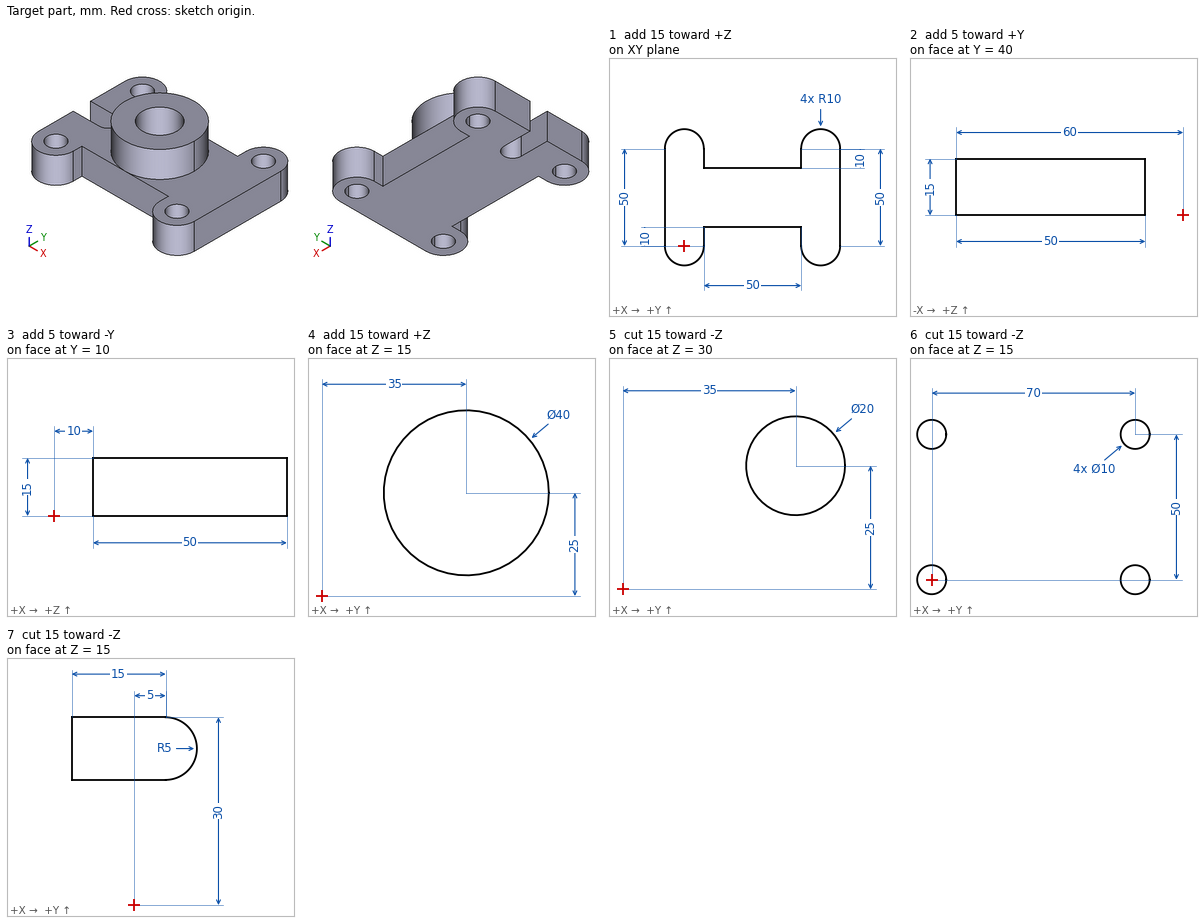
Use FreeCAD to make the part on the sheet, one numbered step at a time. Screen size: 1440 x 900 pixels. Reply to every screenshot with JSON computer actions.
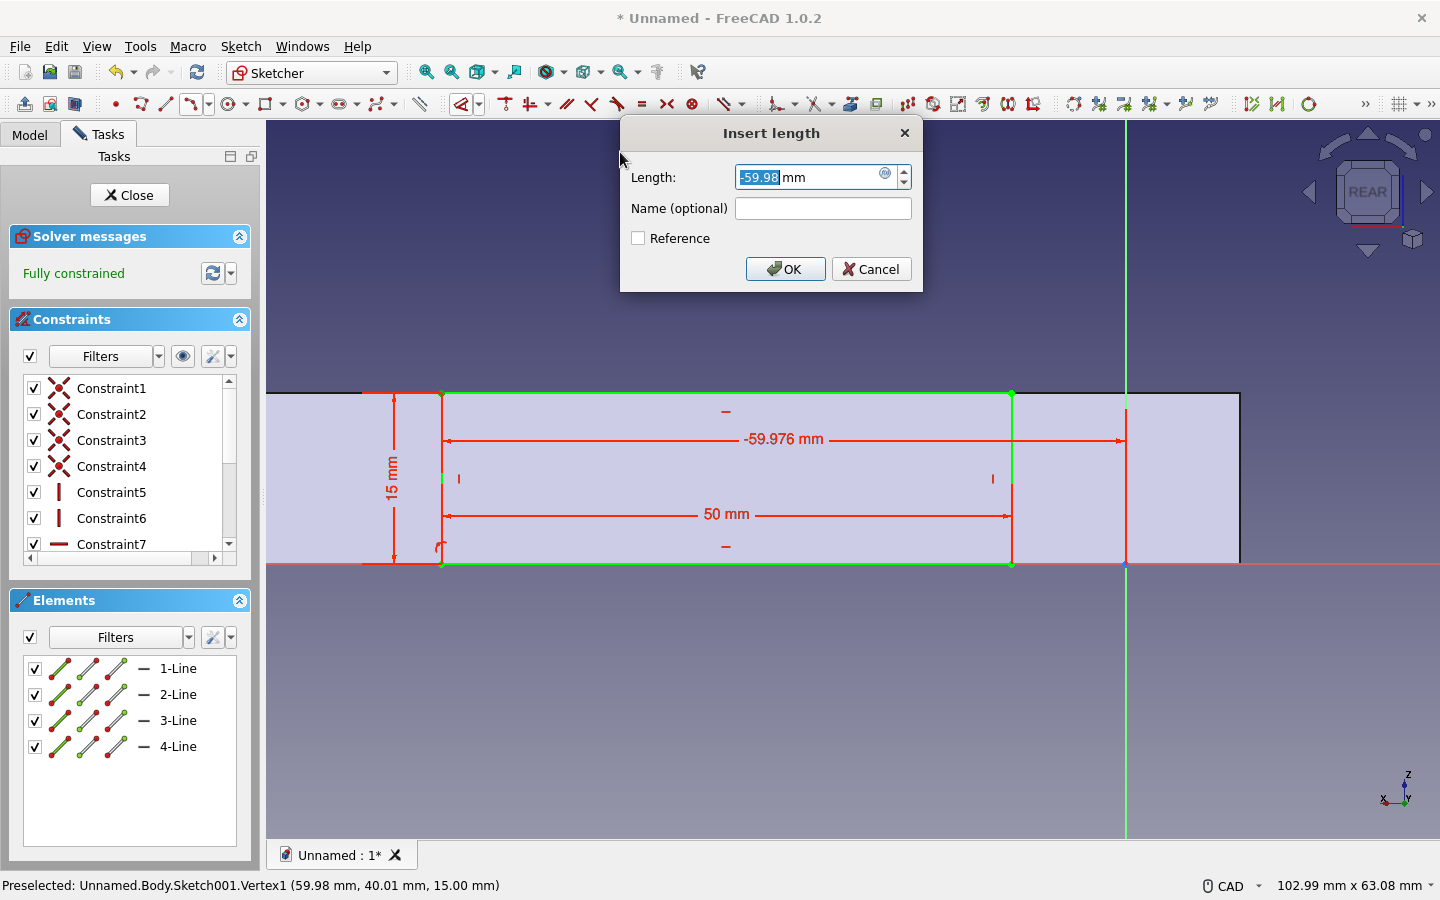
{"action": "type", "text": "-60"}
{"action": "key", "text": "Return"}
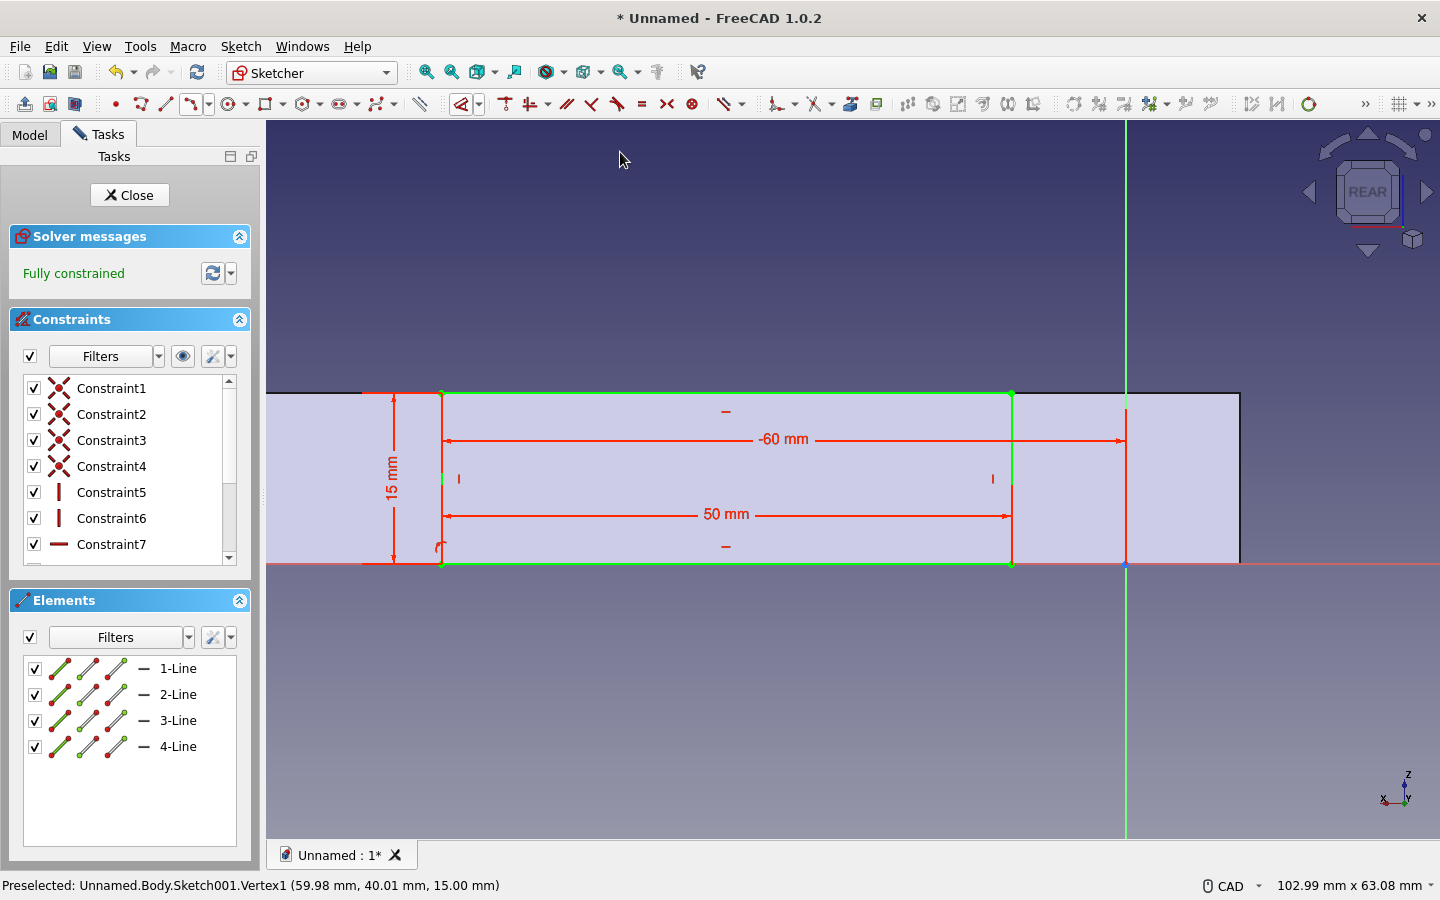
{"action": "left_click", "coordinate": [130, 195]}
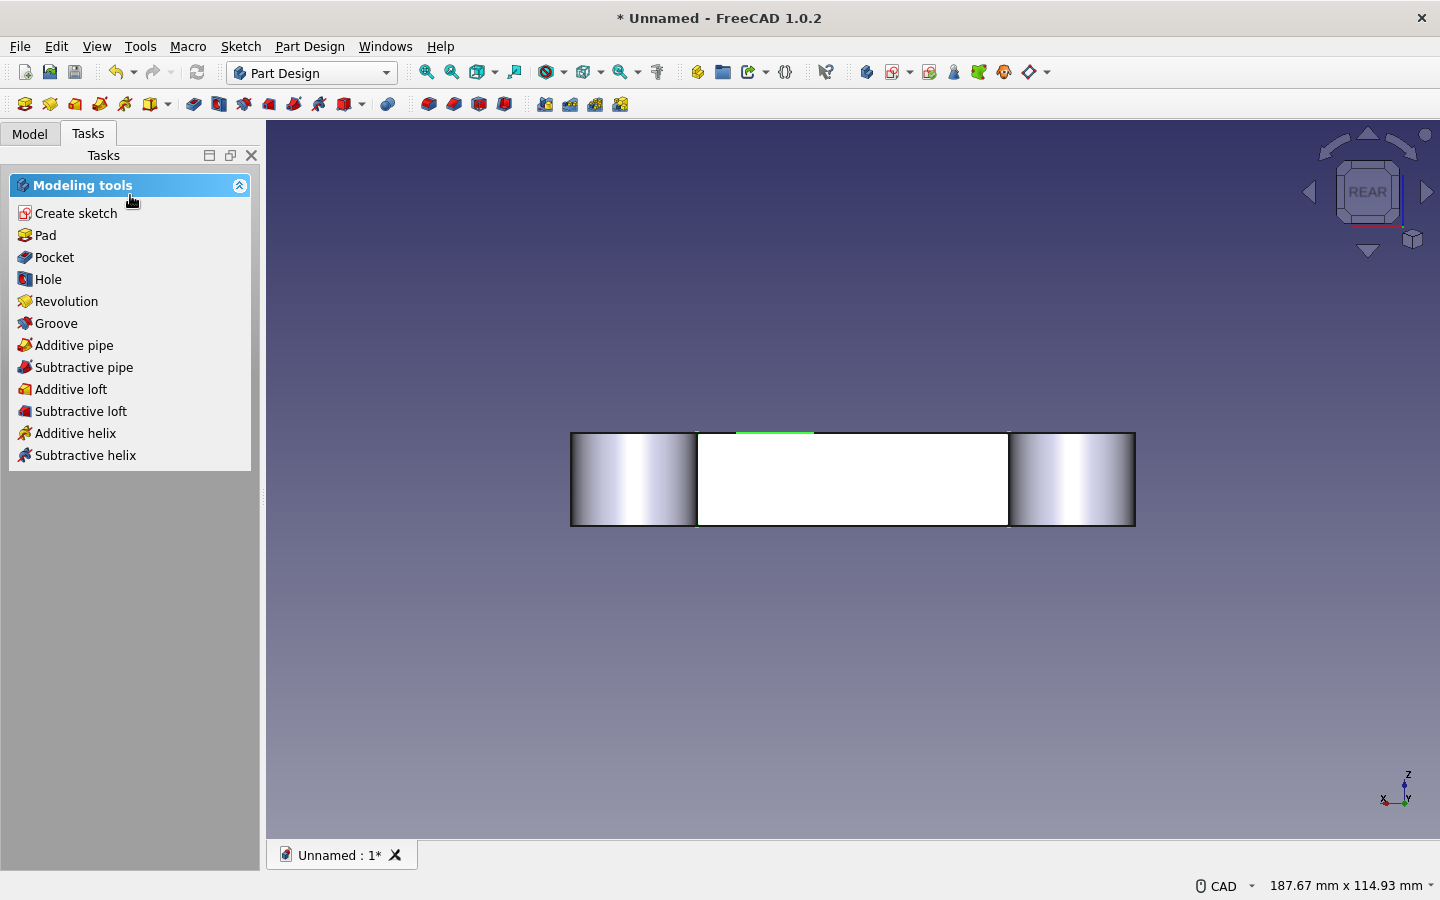
{"action": "left_click", "coordinate": [25, 104]}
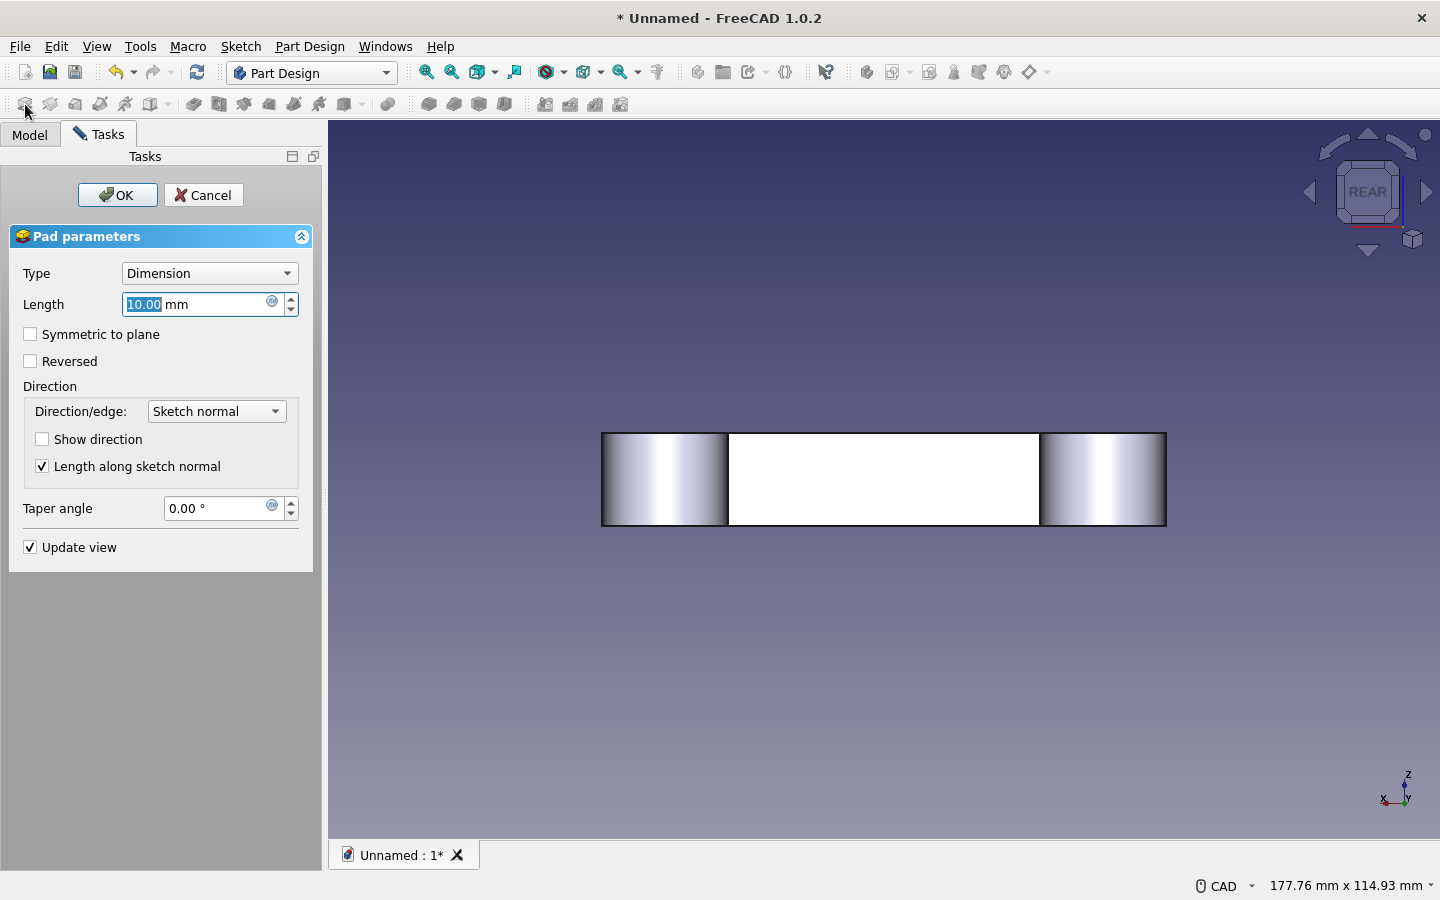
{"action": "type", "text": "5"}
{"action": "key", "text": "Tab"}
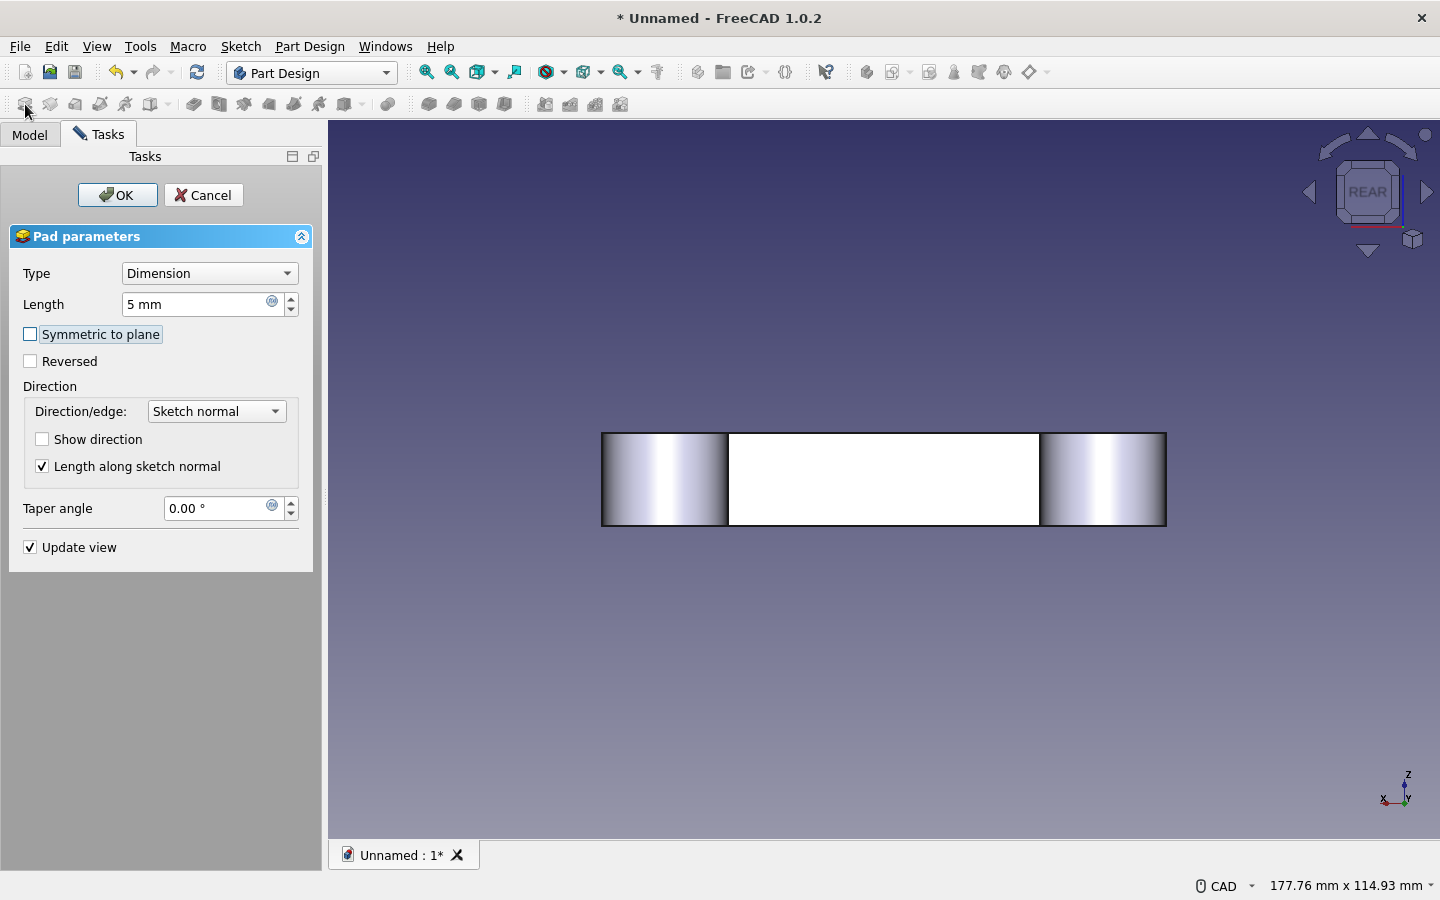
{"action": "left_click", "coordinate": [118, 195]}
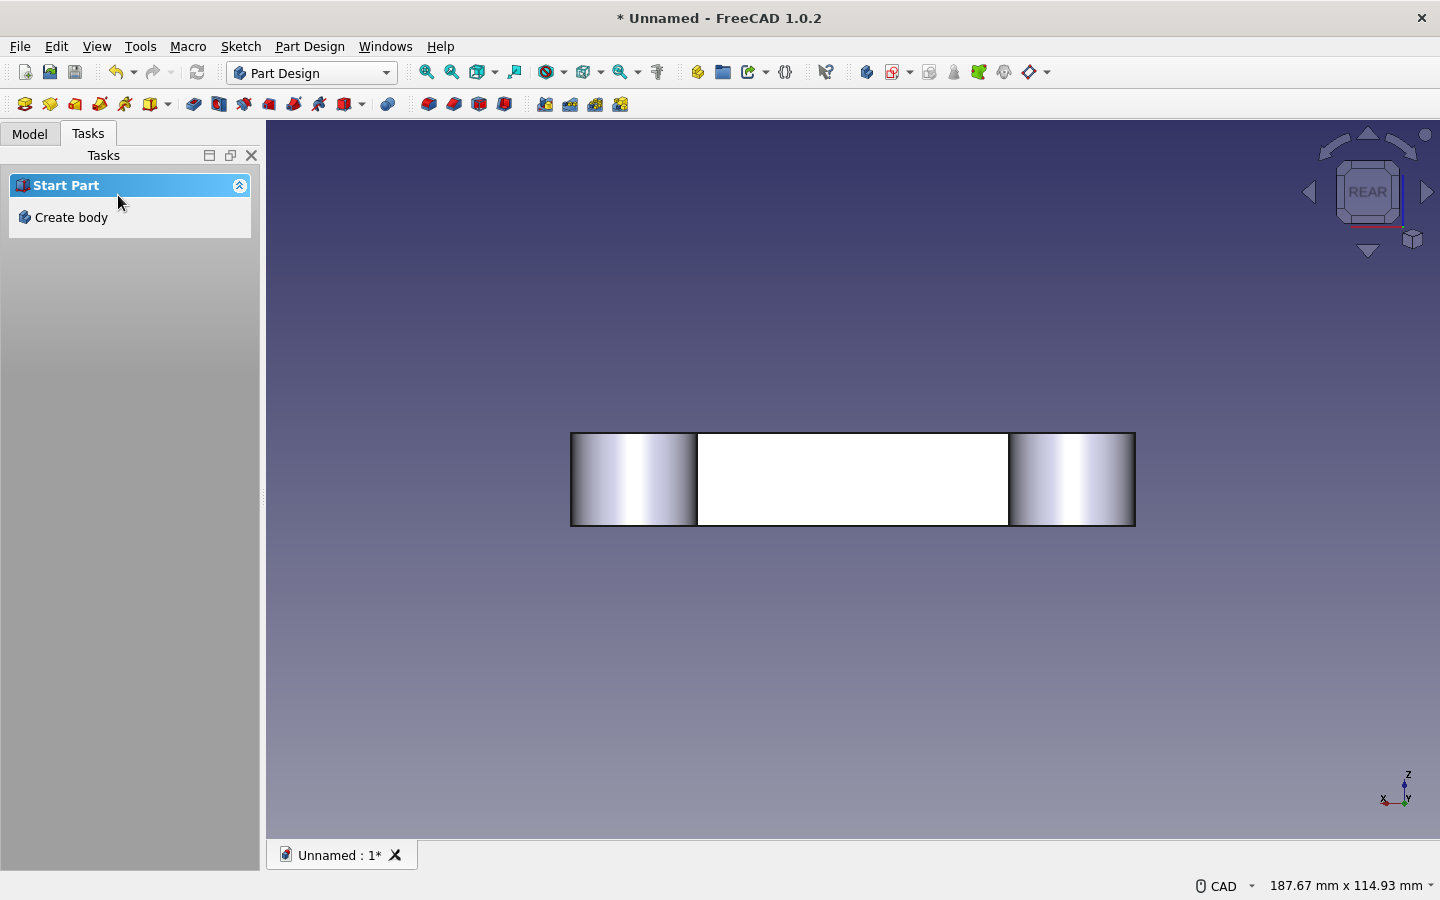
{"action": "key", "text": "0"}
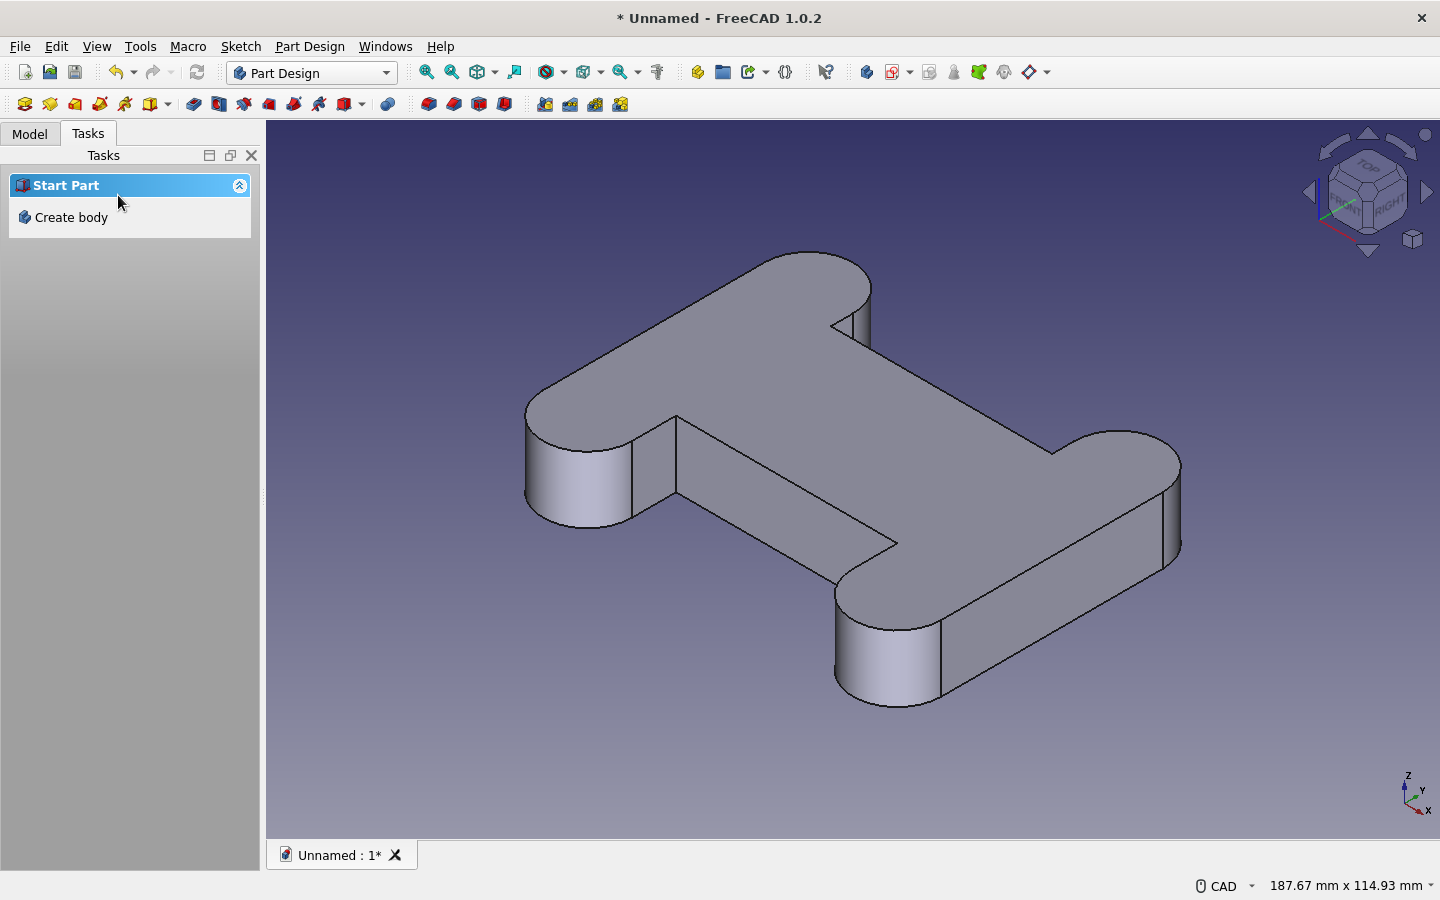
{"action": "left_click", "coordinate": [850, 553]}